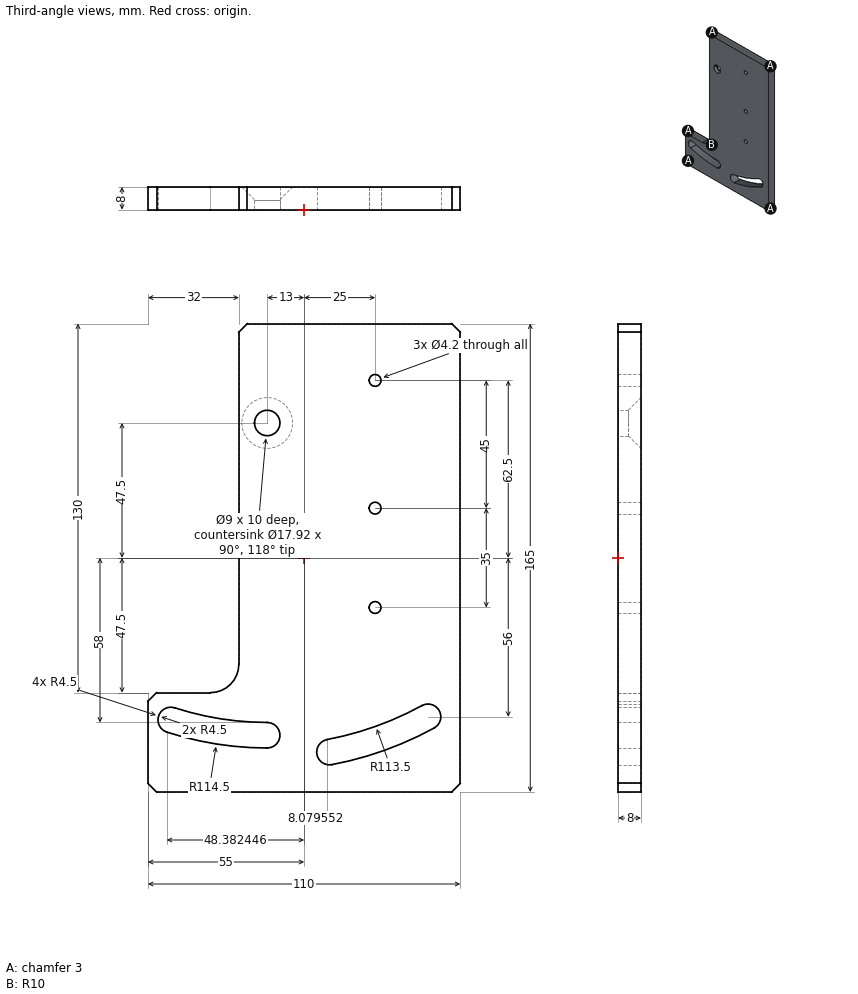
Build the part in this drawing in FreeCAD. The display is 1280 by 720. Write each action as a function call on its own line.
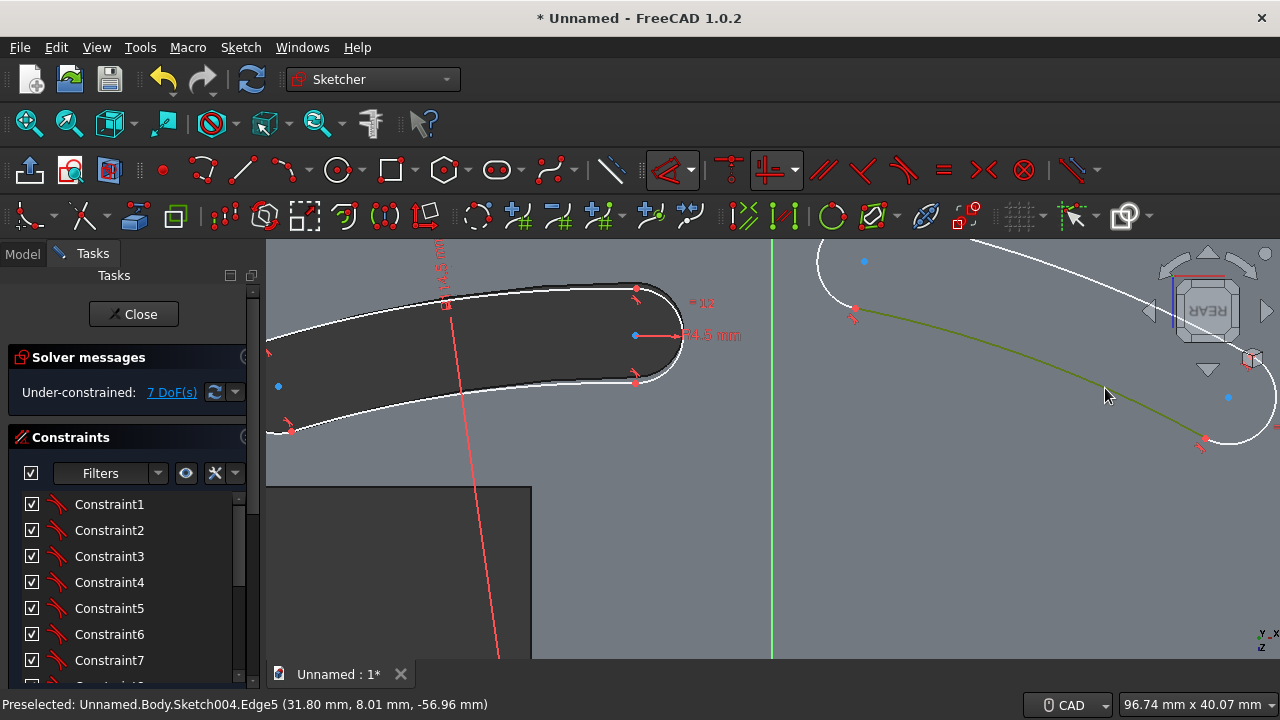
click(694, 170)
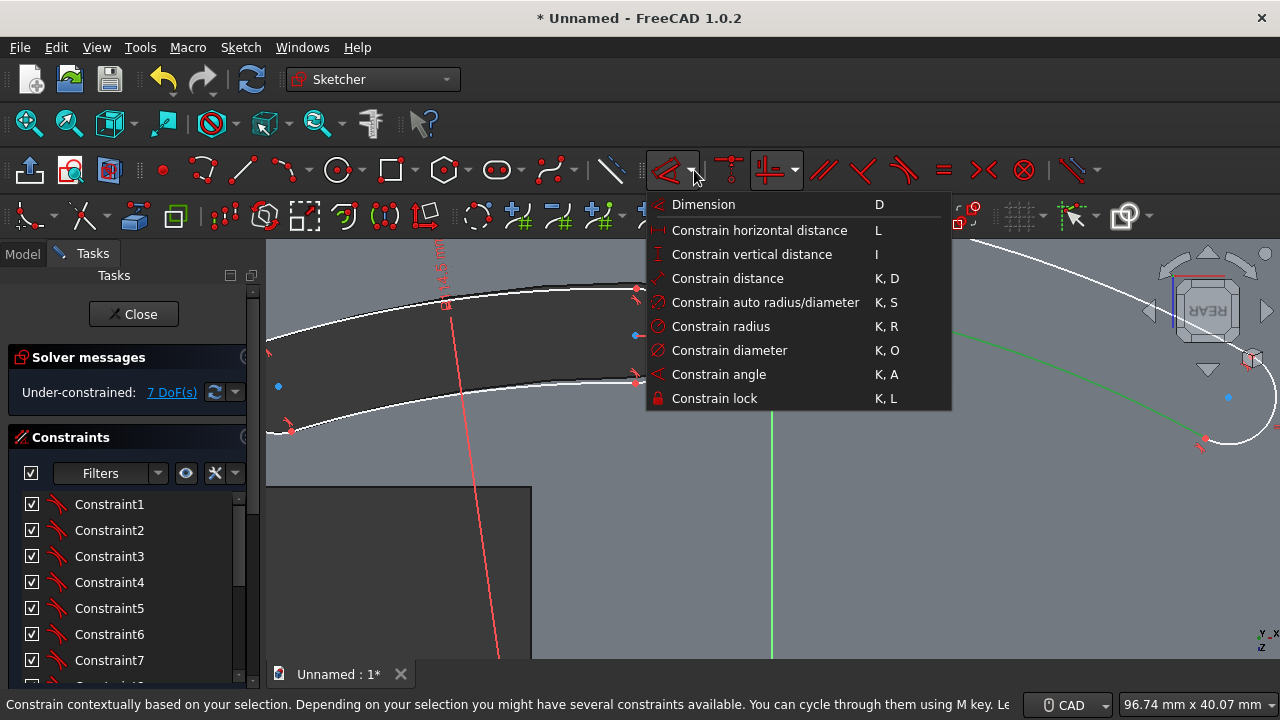
click(799, 326)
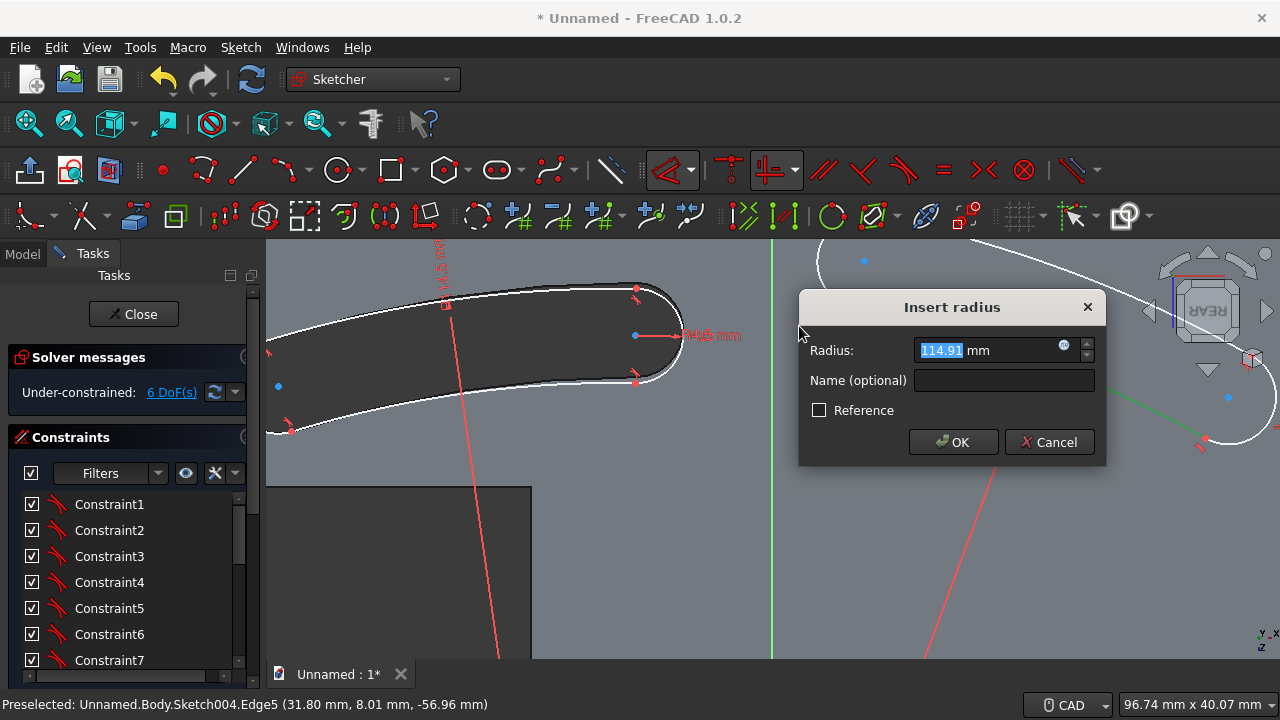
text(113.5)
key(Return)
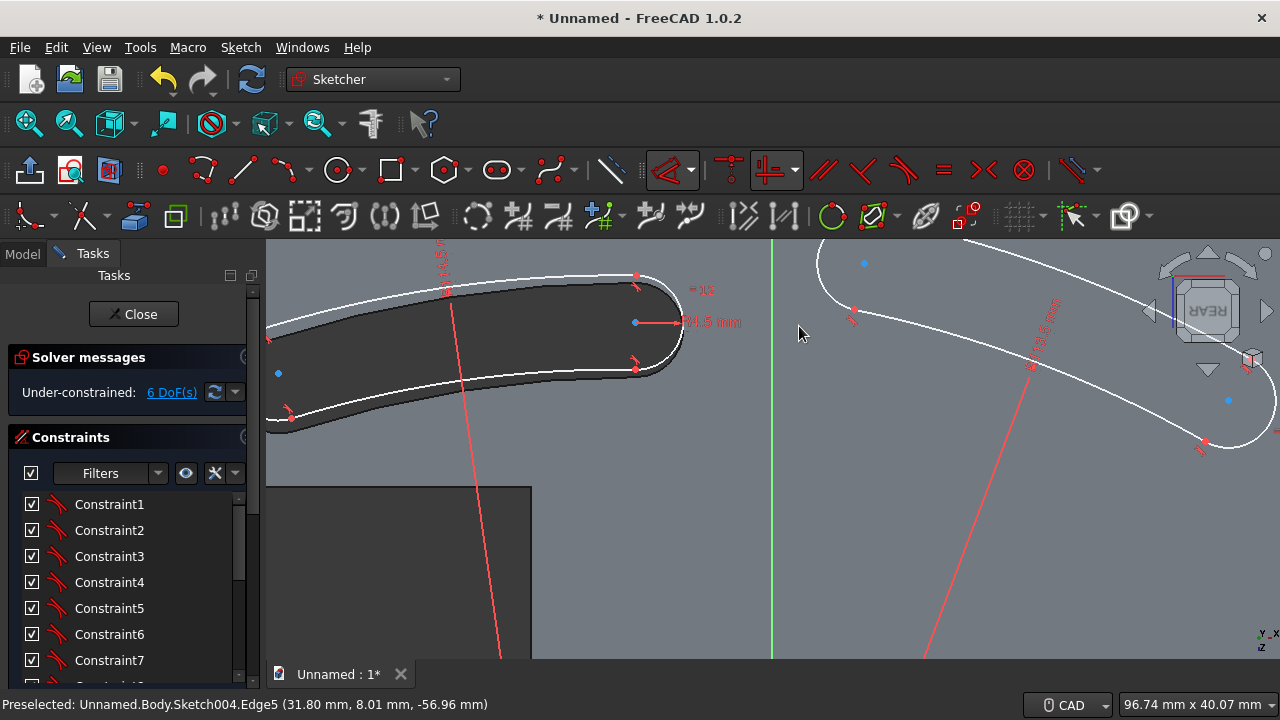
click(635, 370)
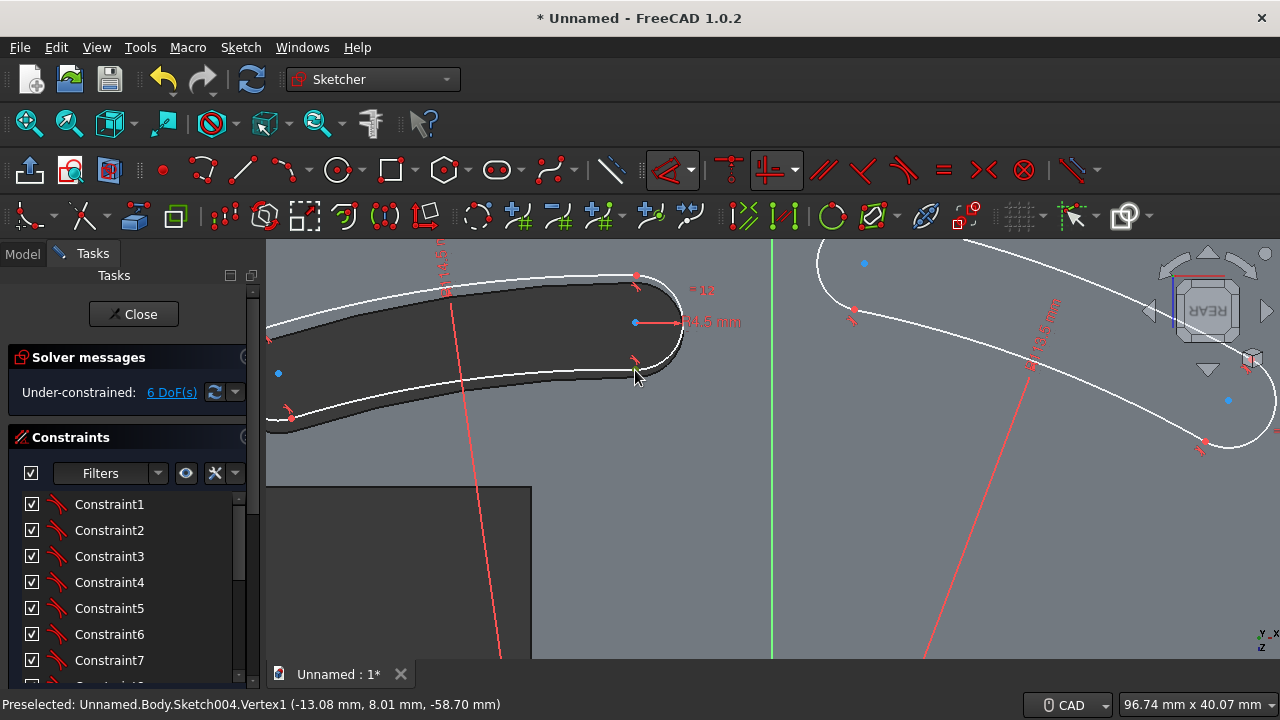
key(l)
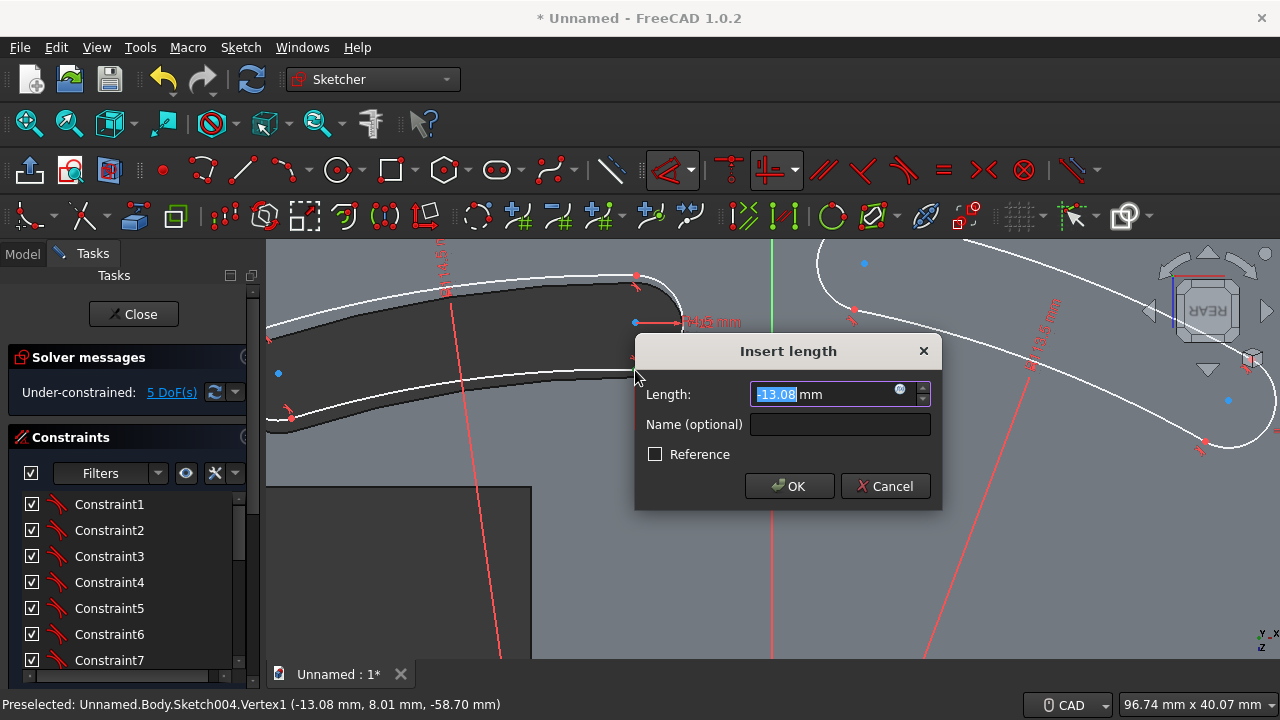
text(-13)
key(Return)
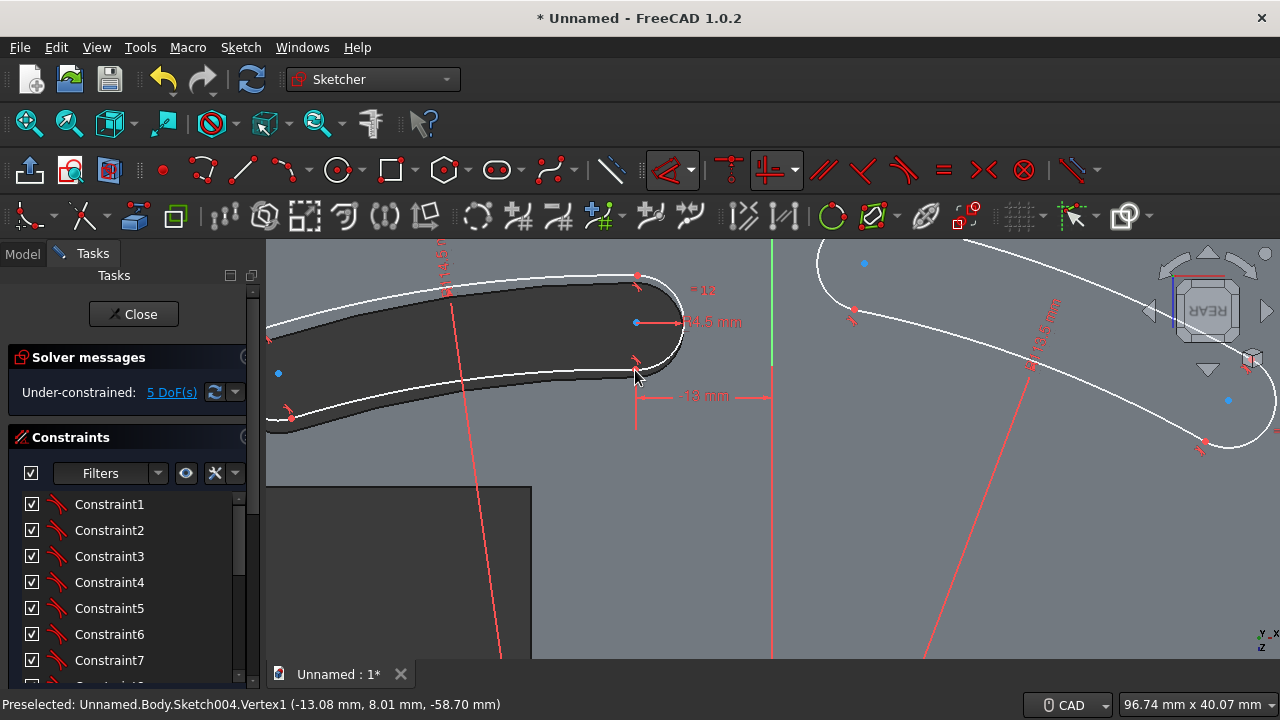
click(636, 370)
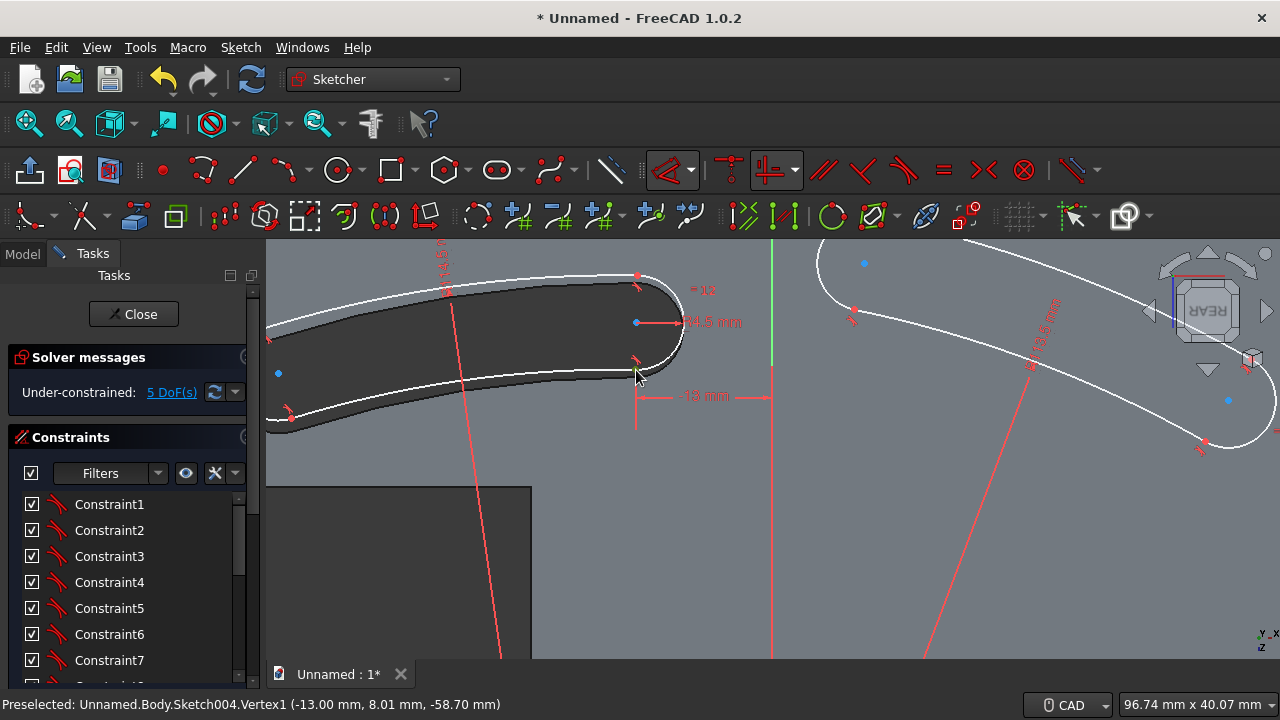
click(694, 170)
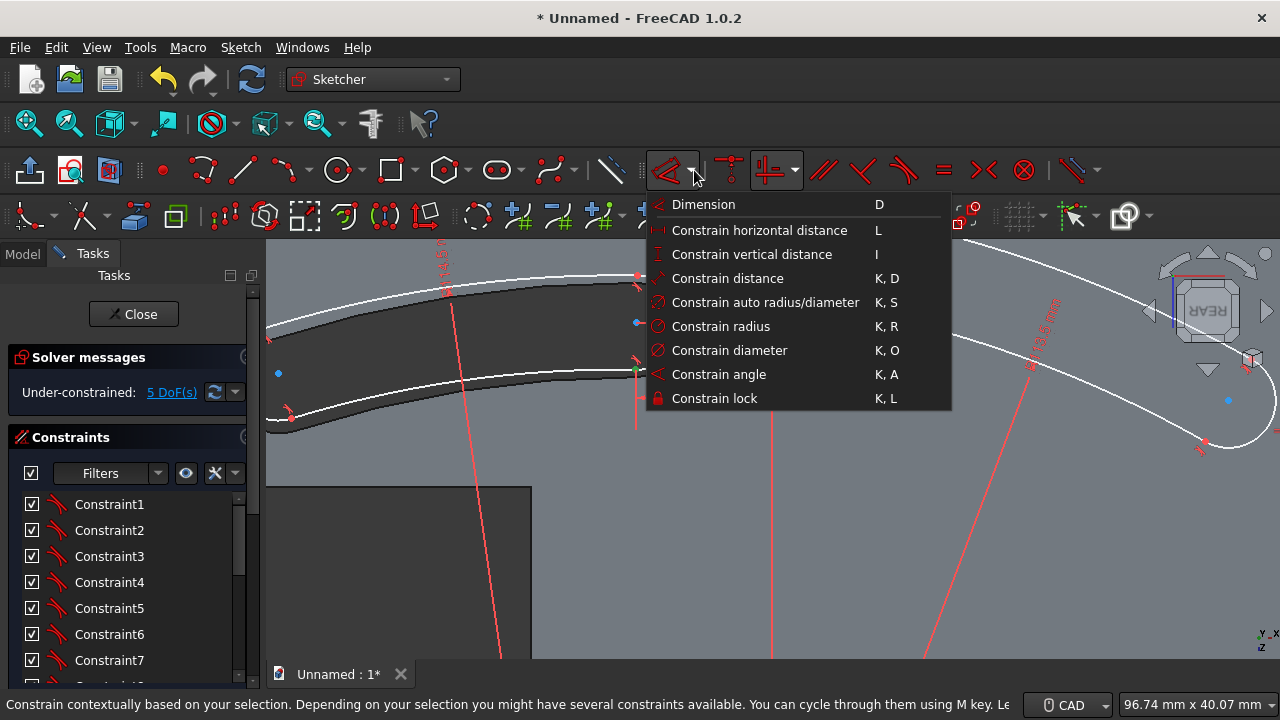
click(799, 254)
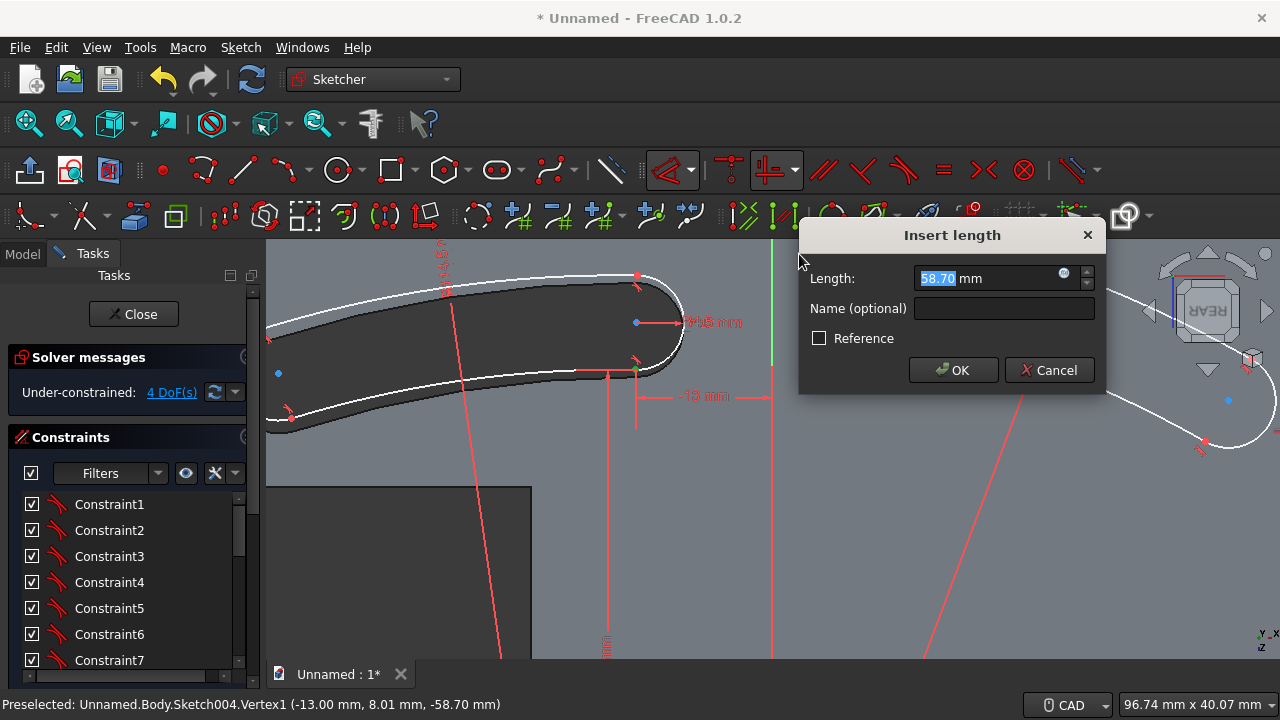
text(58)
key(Return)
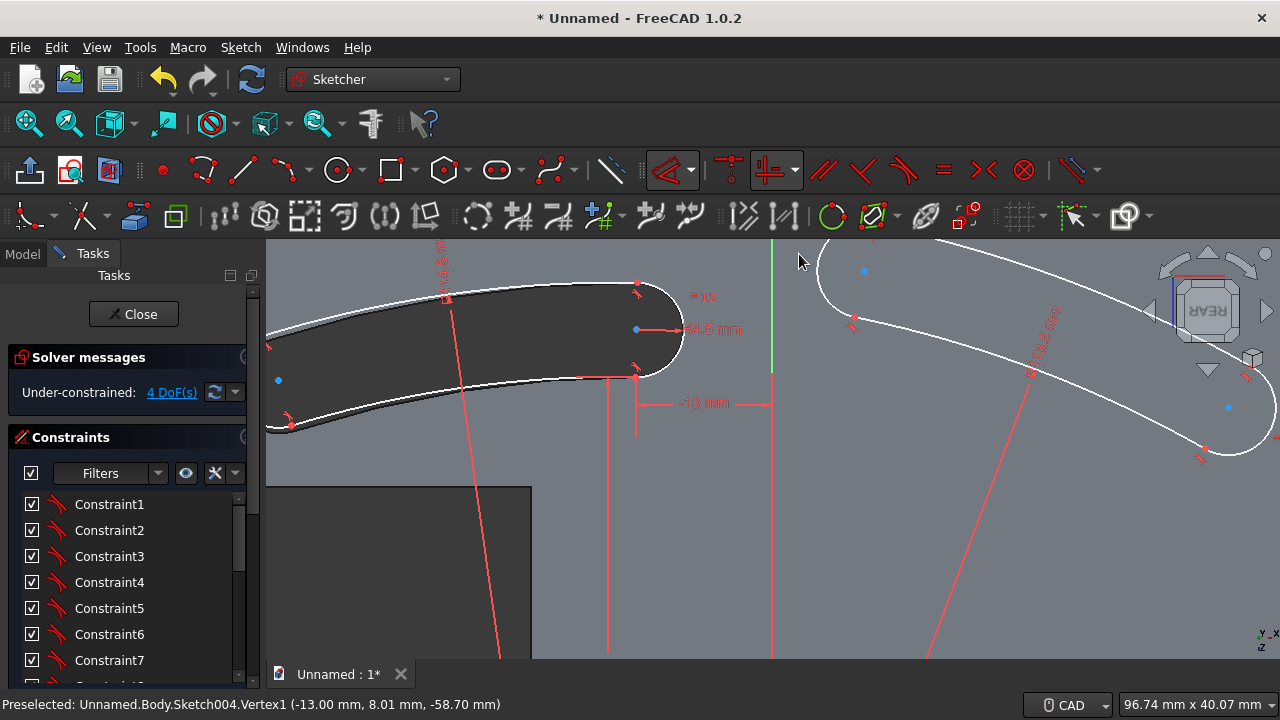
scroll(676, 359, down, 5)